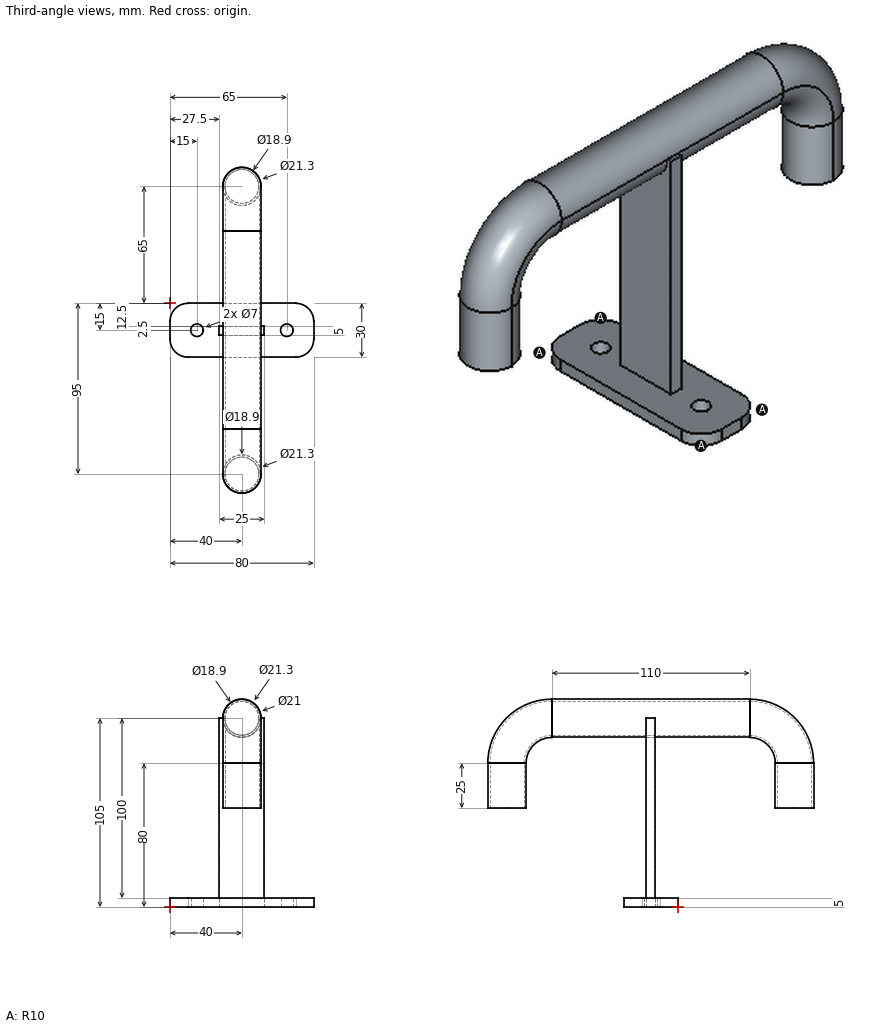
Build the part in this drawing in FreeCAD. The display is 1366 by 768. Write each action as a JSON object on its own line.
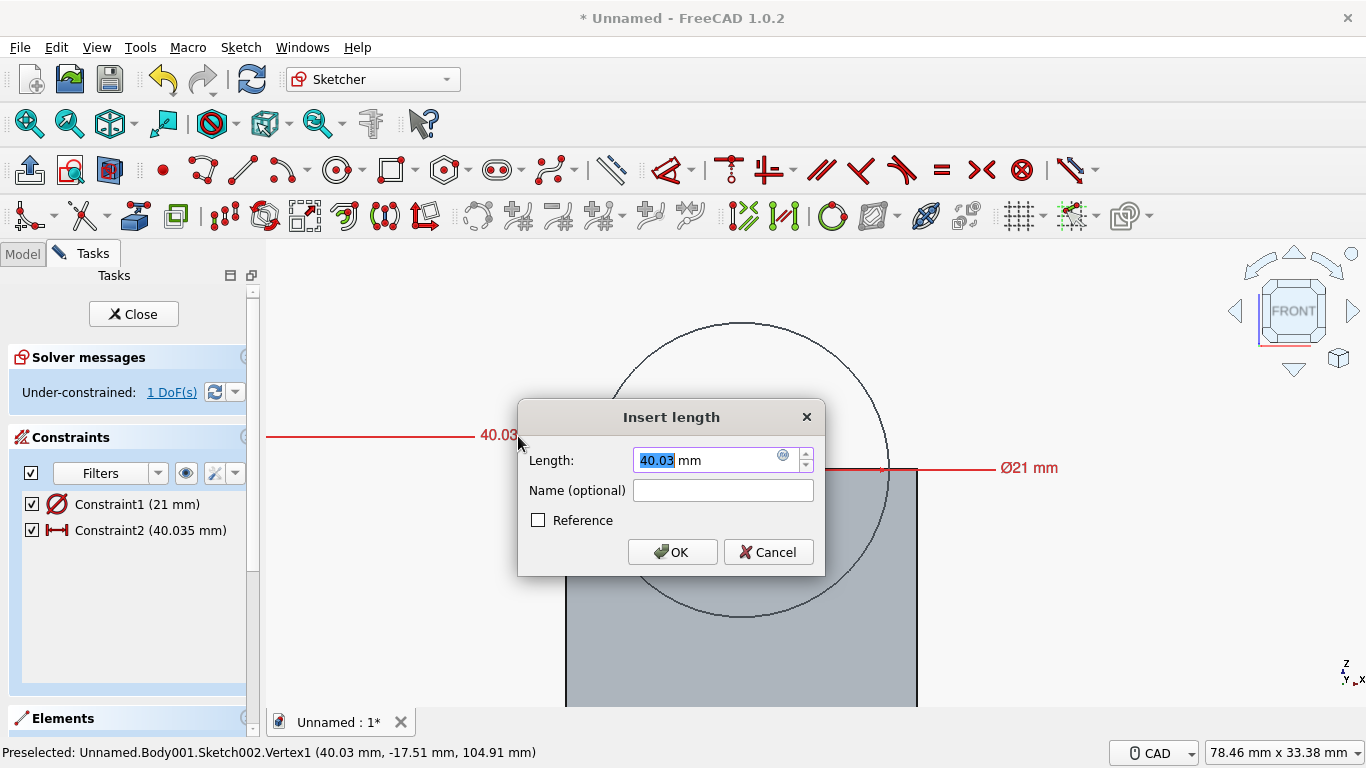
{"action": "type", "text": "40"}
{"action": "key", "text": "Return"}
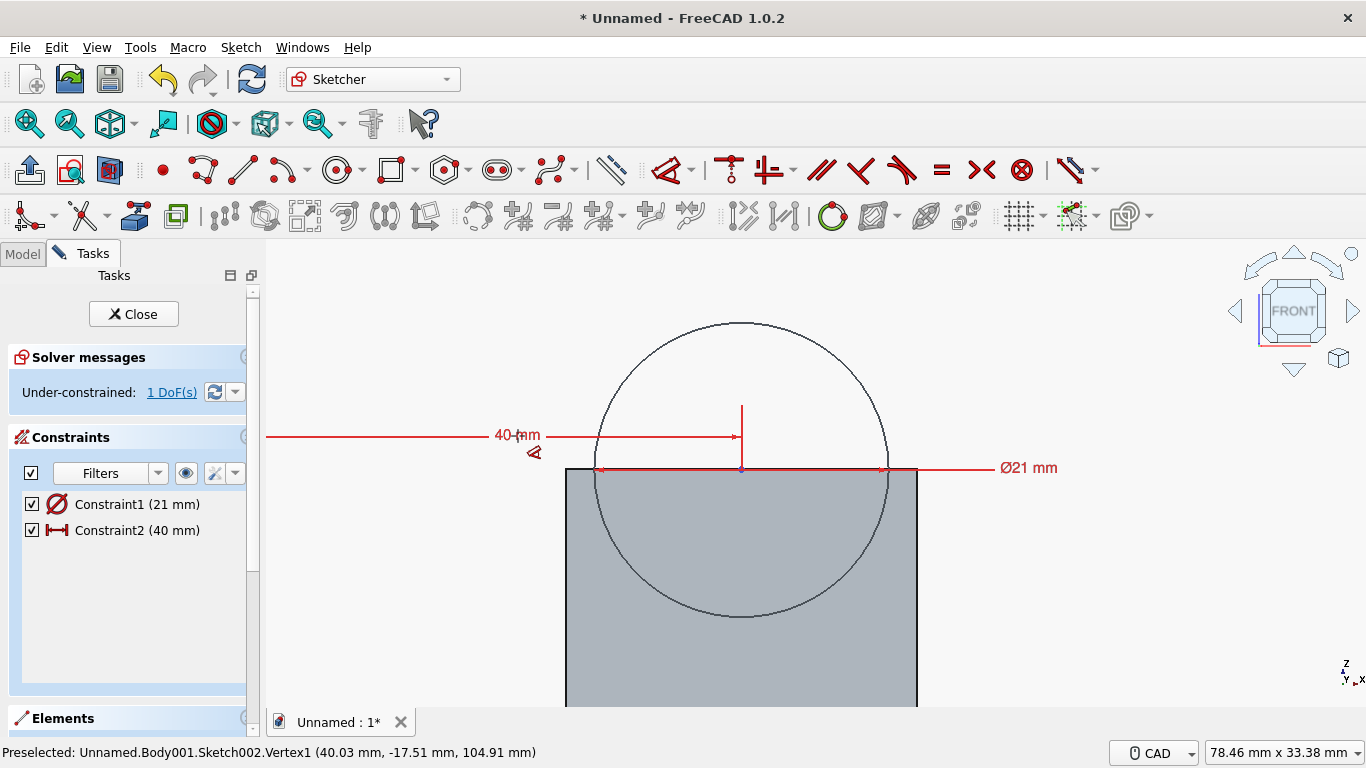
{"action": "left_click", "coordinate": [742, 470]}
{"action": "left_click", "coordinate": [776, 575]}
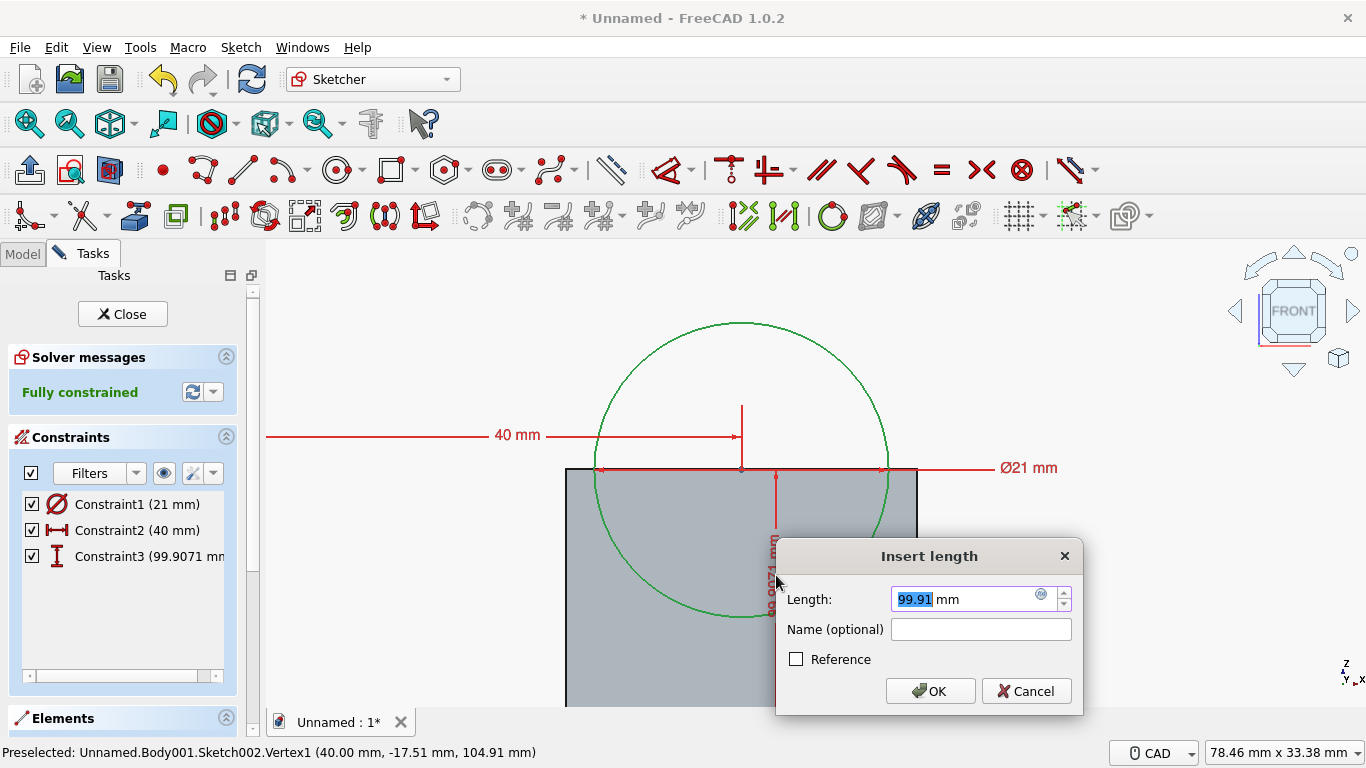
{"action": "type", "text": "100"}
{"action": "key", "text": "Return"}
{"action": "key", "text": "Escape"}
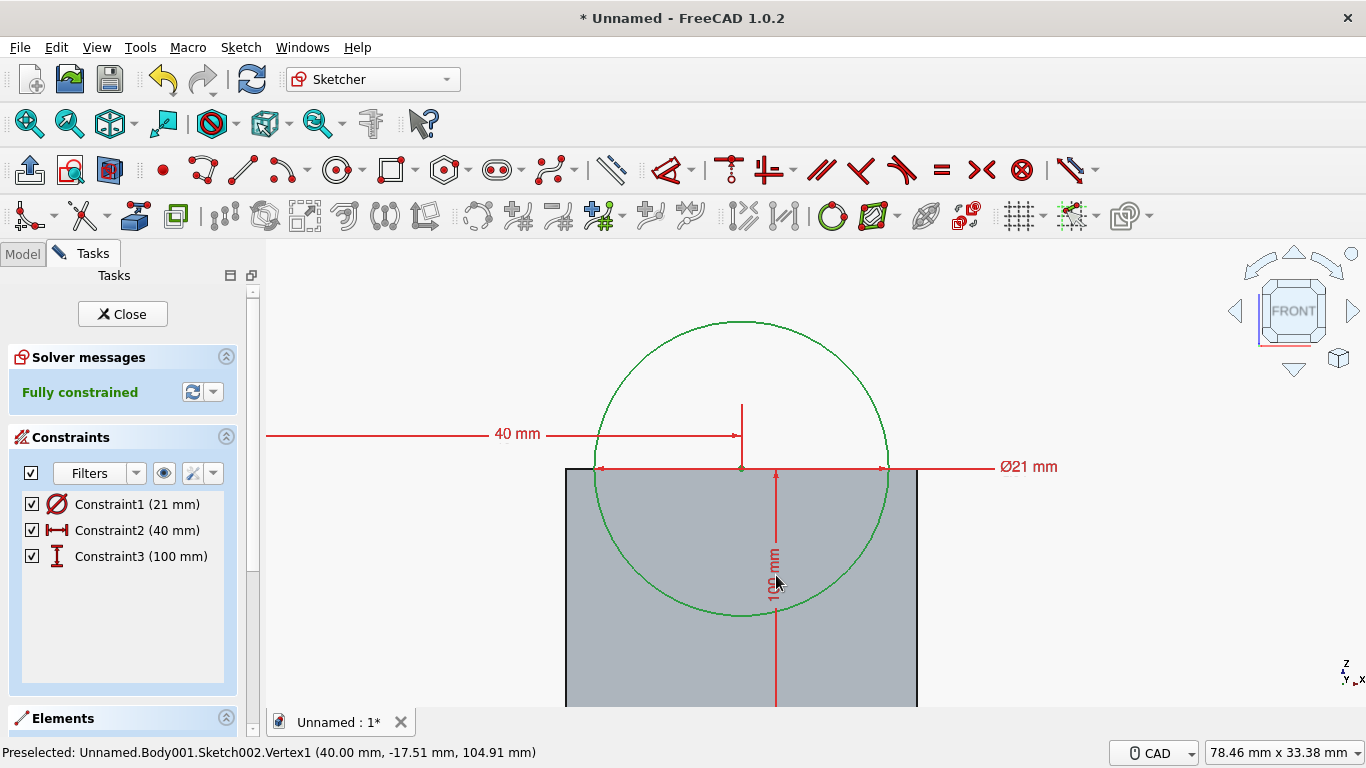
{"action": "left_click", "coordinate": [123, 314]}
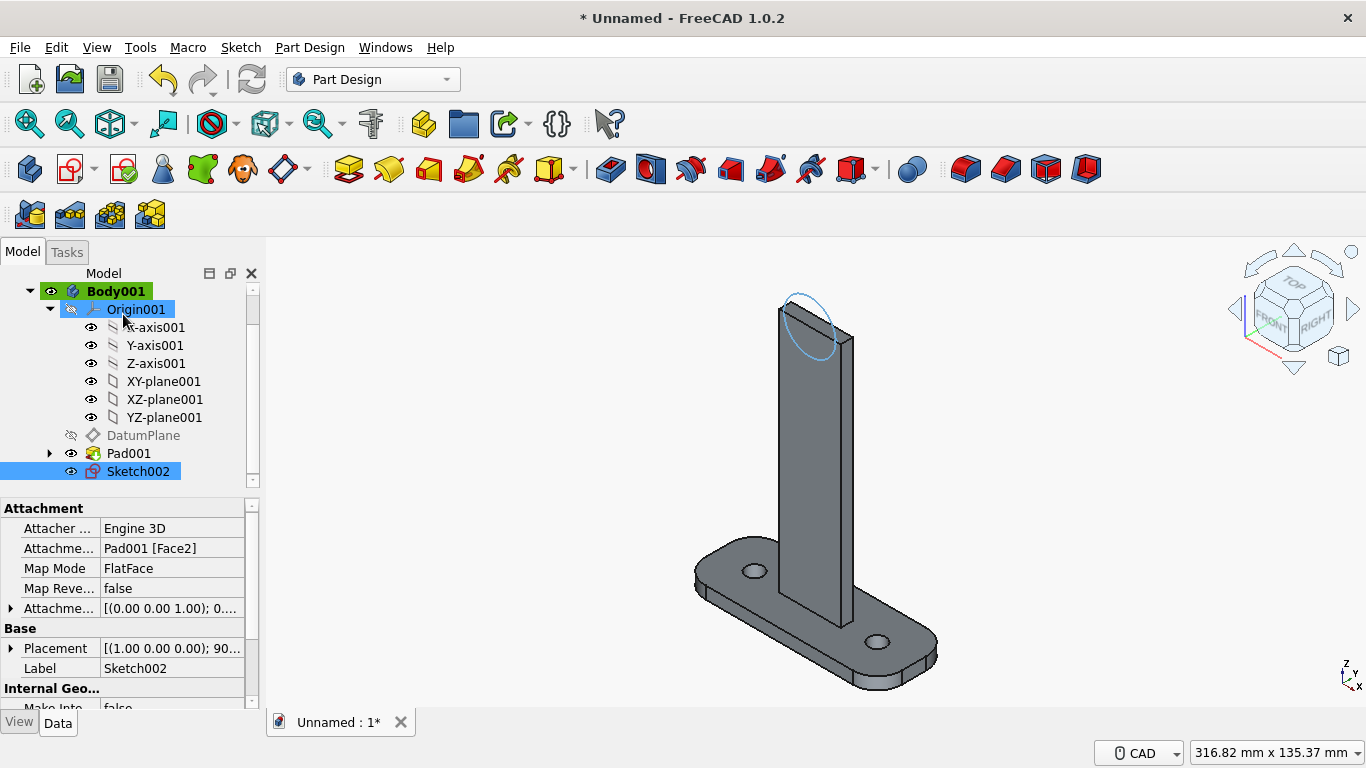
{"action": "left_click", "coordinate": [612, 170]}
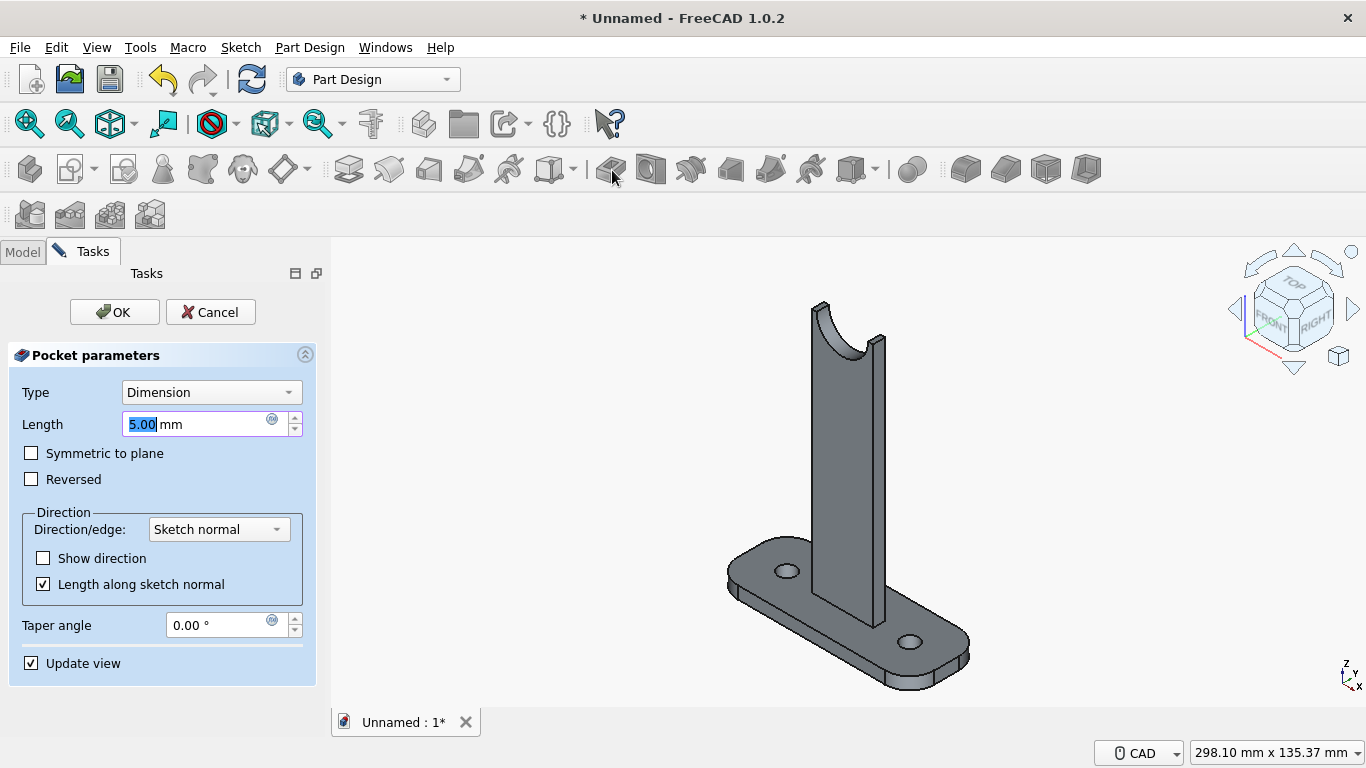
{"action": "left_click", "coordinate": [212, 392]}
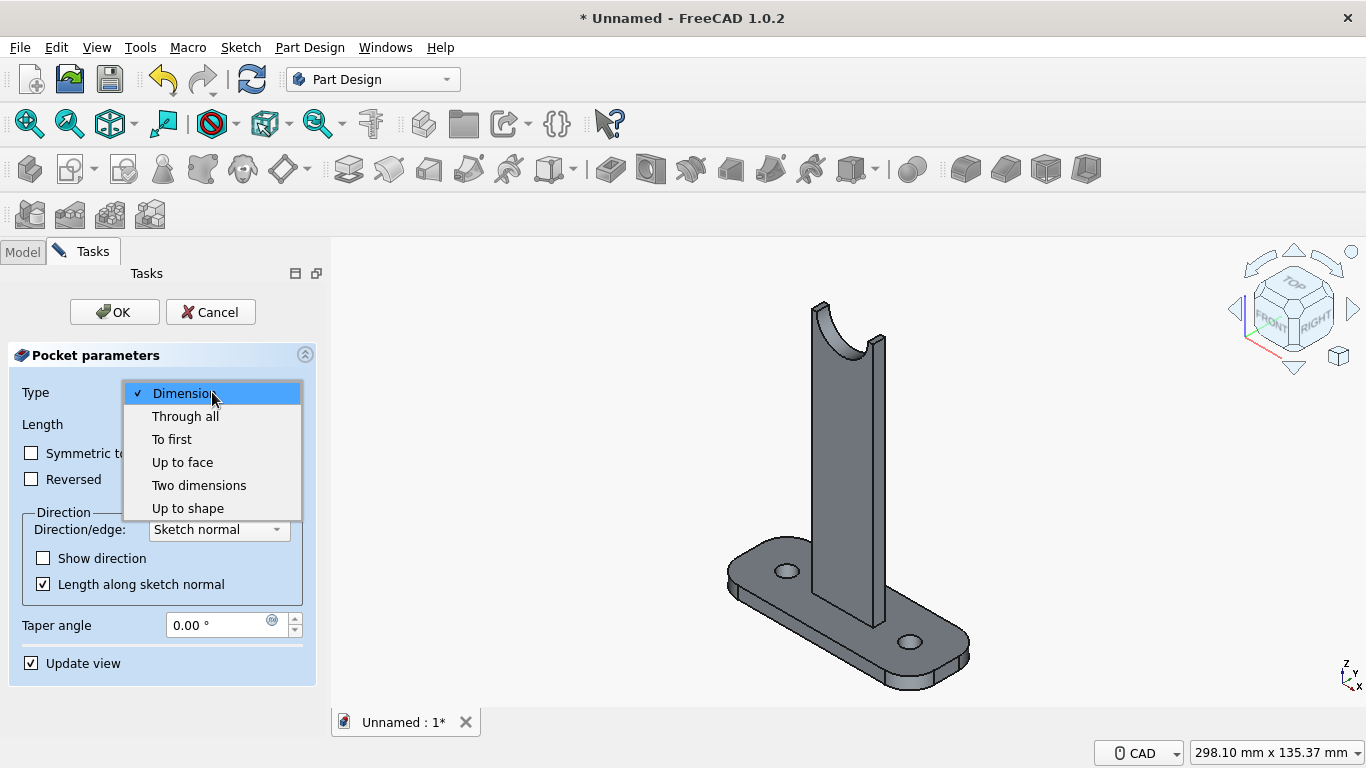
{"action": "left_click", "coordinate": [212, 416]}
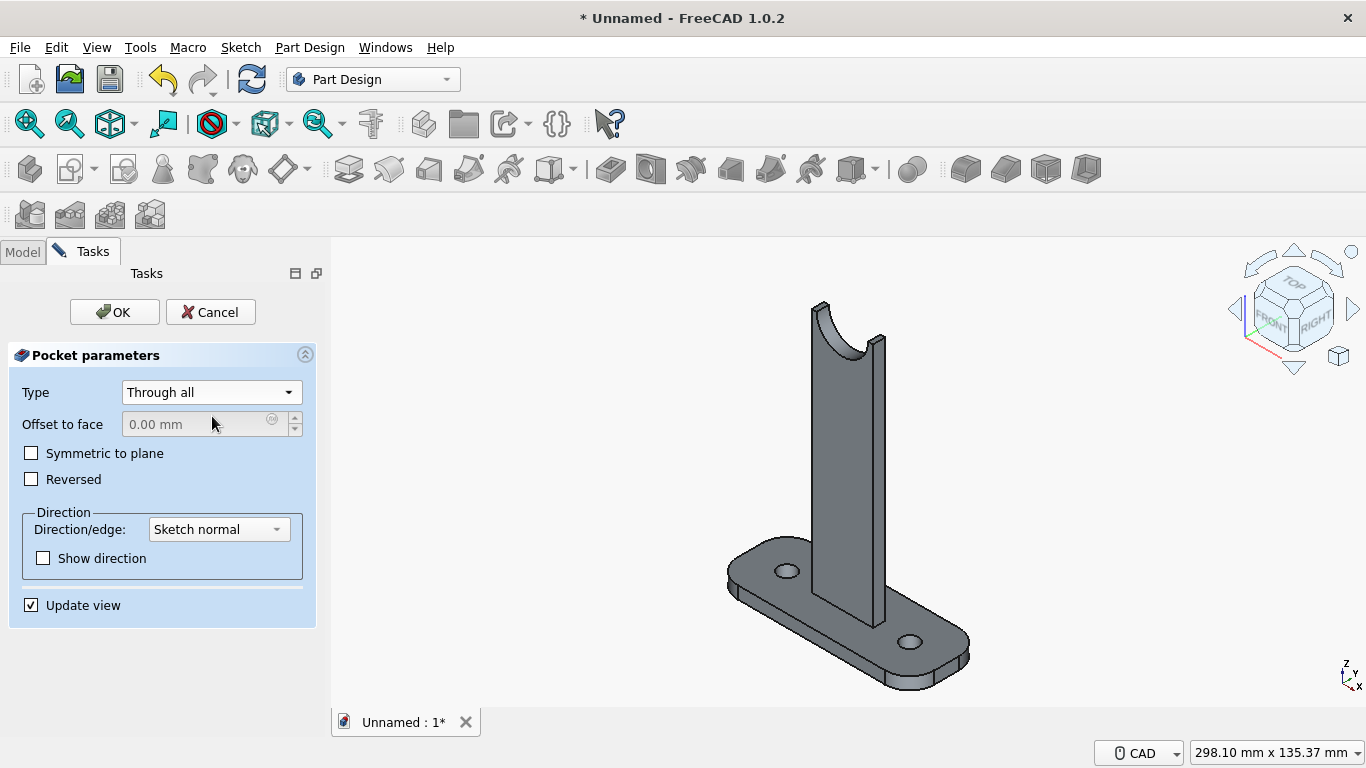
{"action": "left_click", "coordinate": [115, 312]}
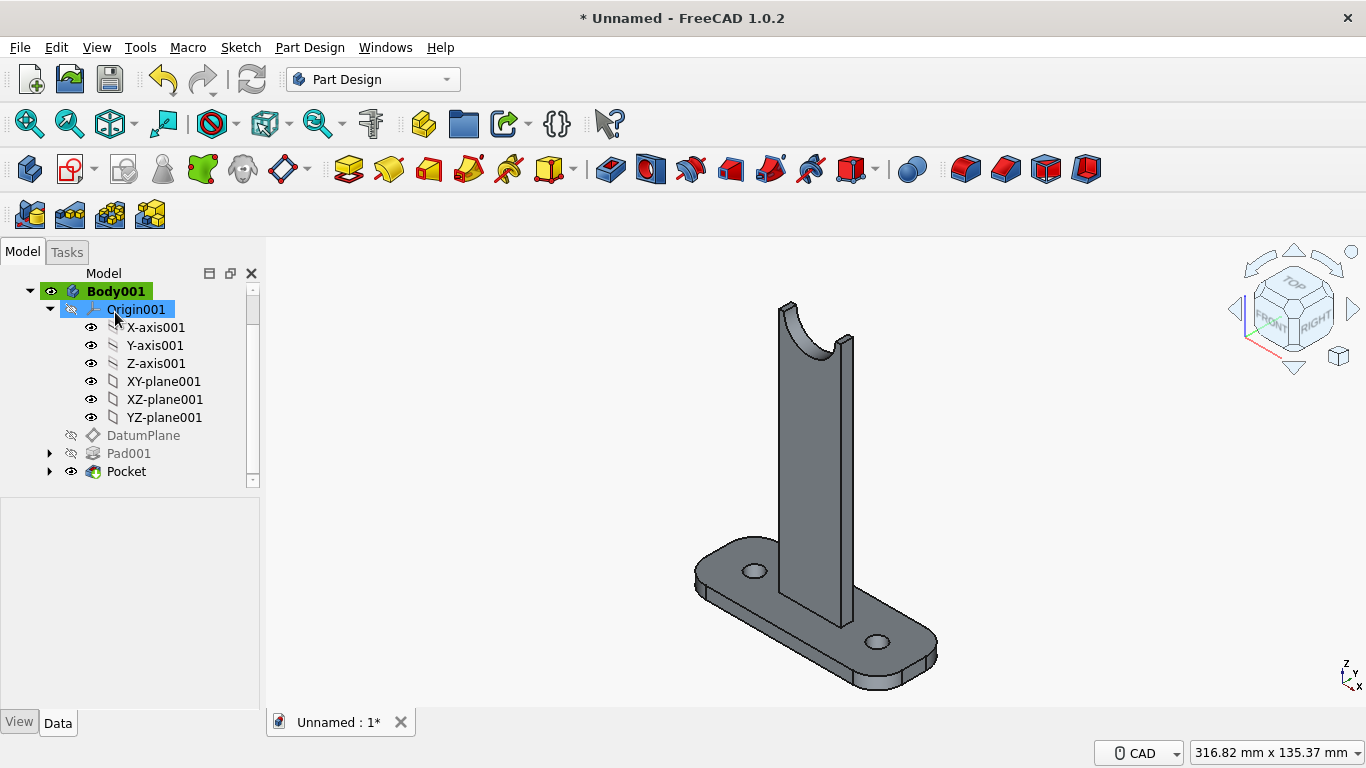
{"action": "left_click", "coordinate": [30, 170]}